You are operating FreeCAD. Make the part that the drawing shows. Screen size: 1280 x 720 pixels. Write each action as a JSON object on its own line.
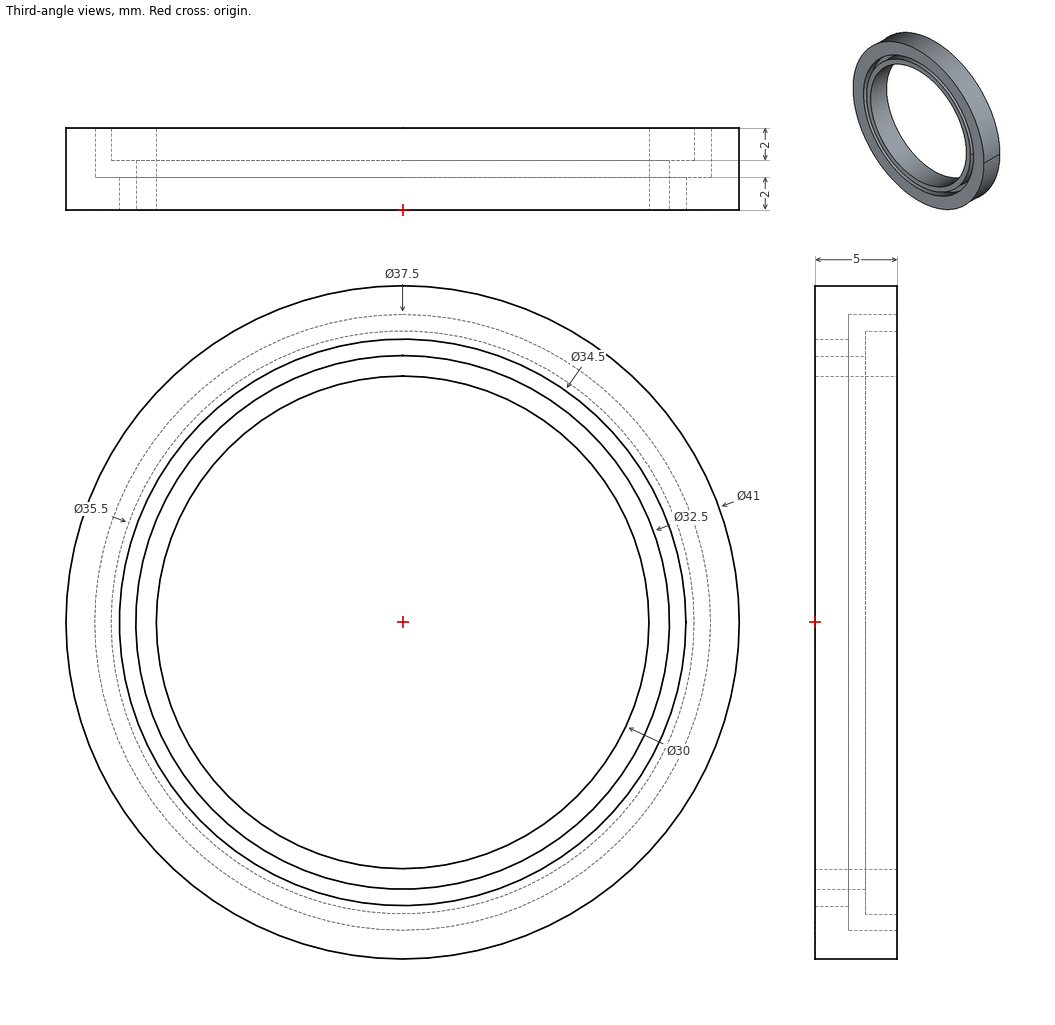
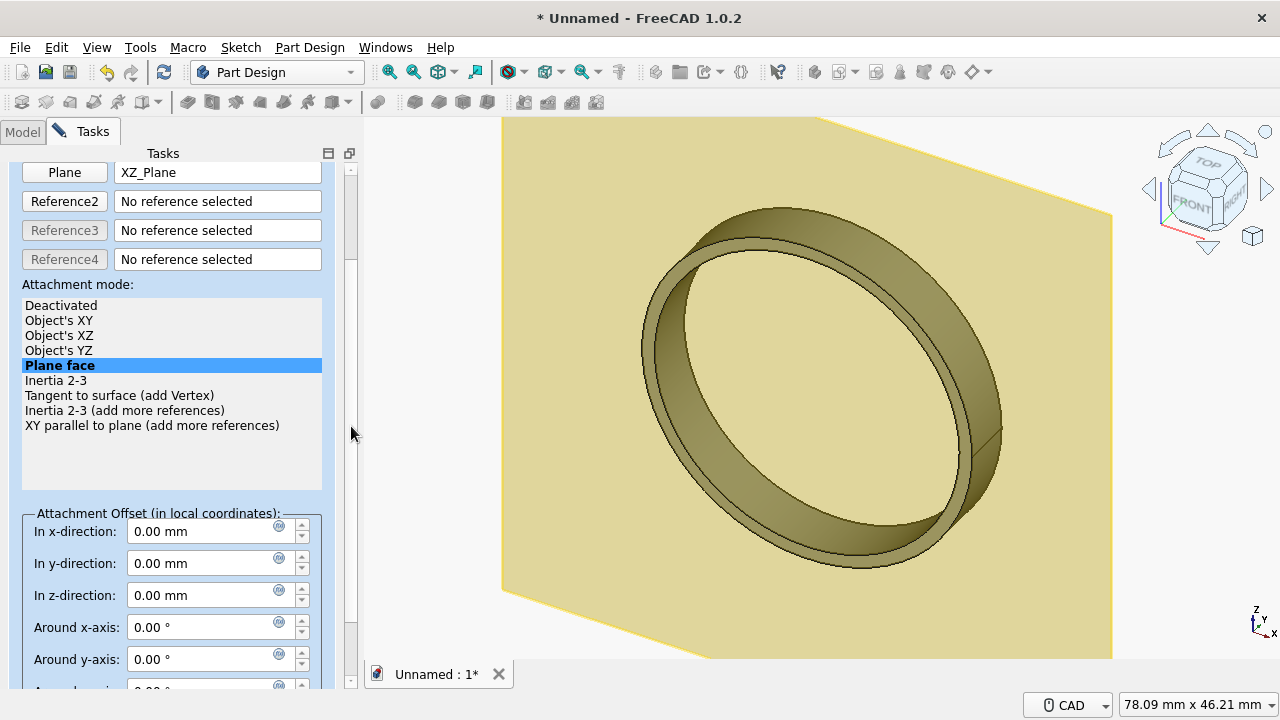
{"action": "triple_click", "coordinate": [210, 595]}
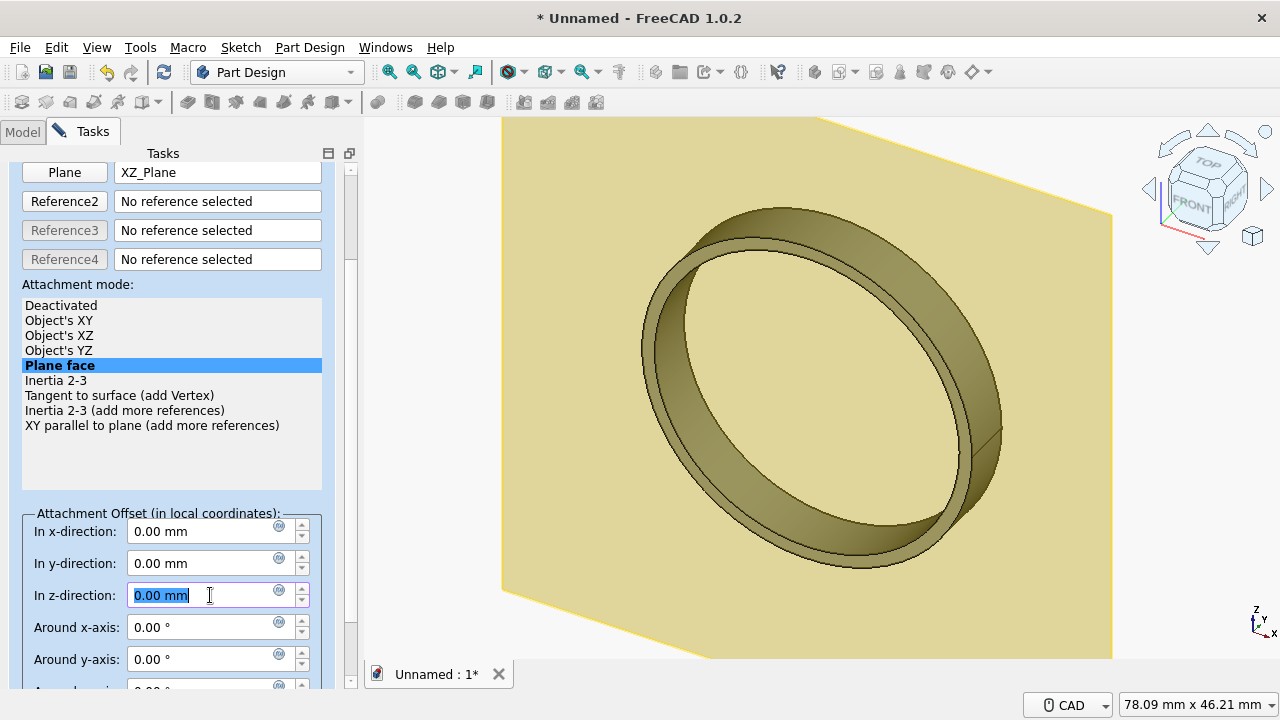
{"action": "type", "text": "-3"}
{"action": "key", "text": "Tab"}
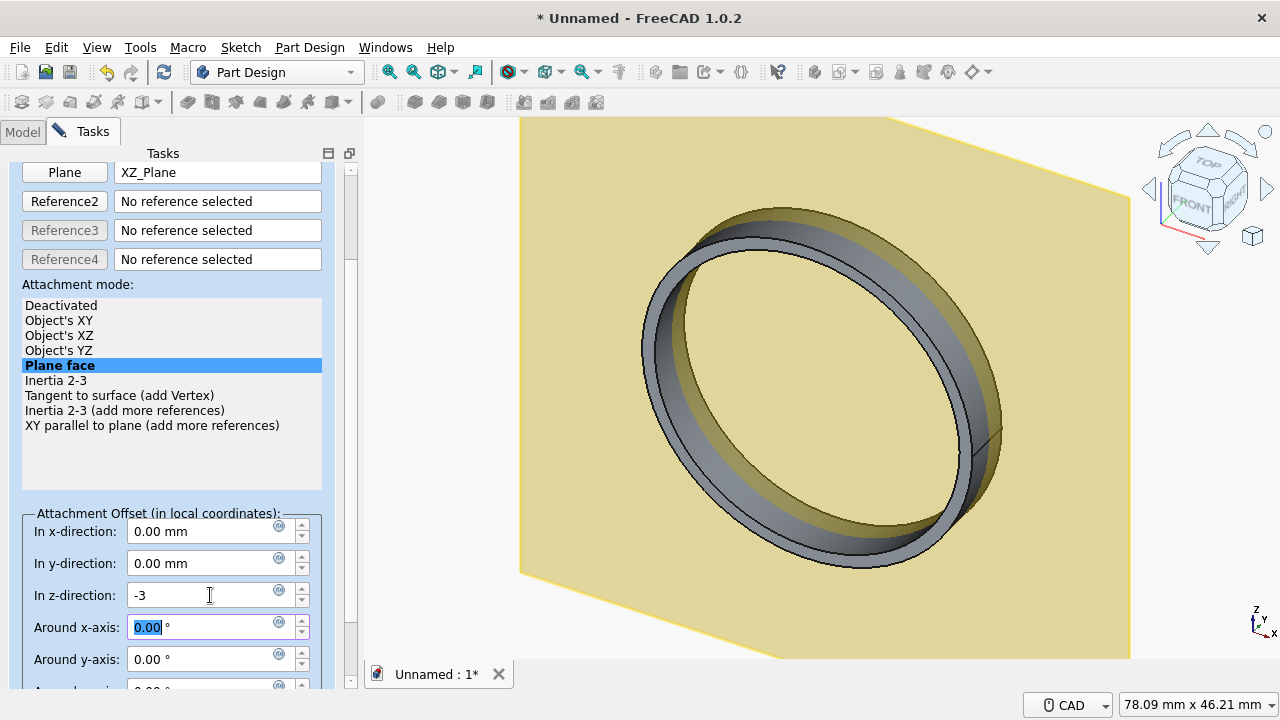
{"action": "scroll", "coordinate": [351, 426], "scroll_direction": "up", "scroll_amount": 3}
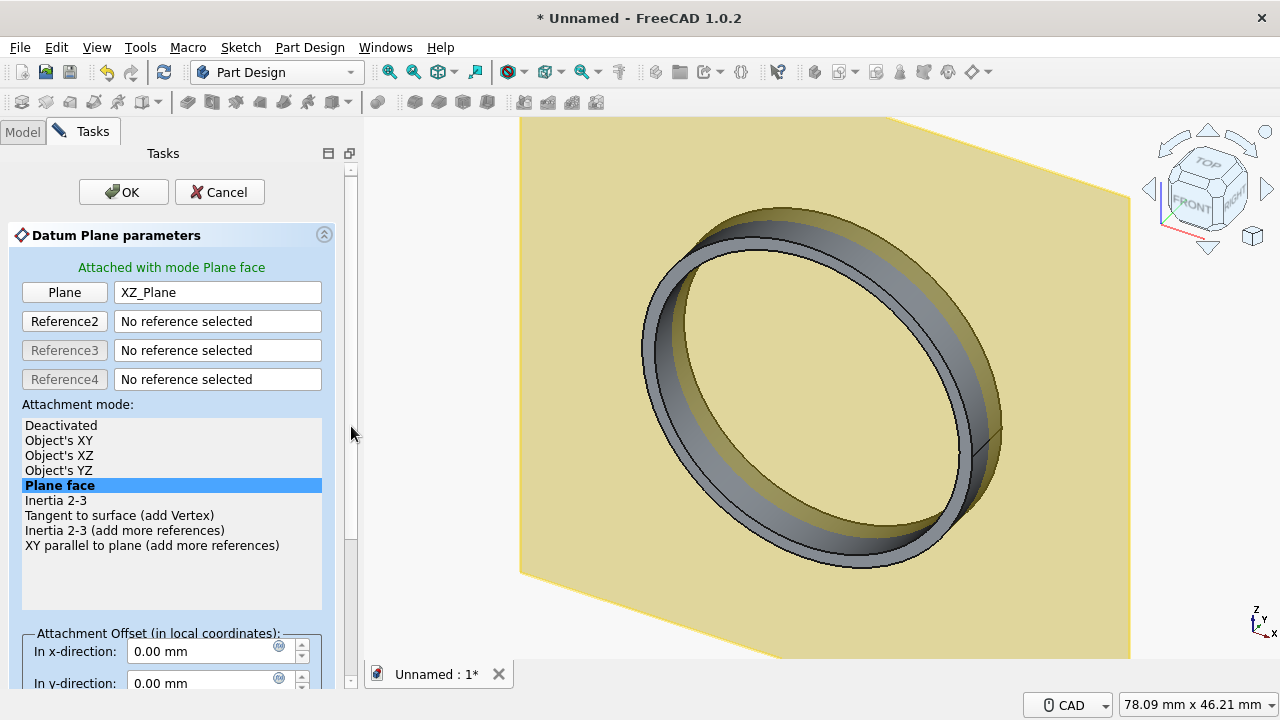
{"action": "left_click", "coordinate": [124, 192]}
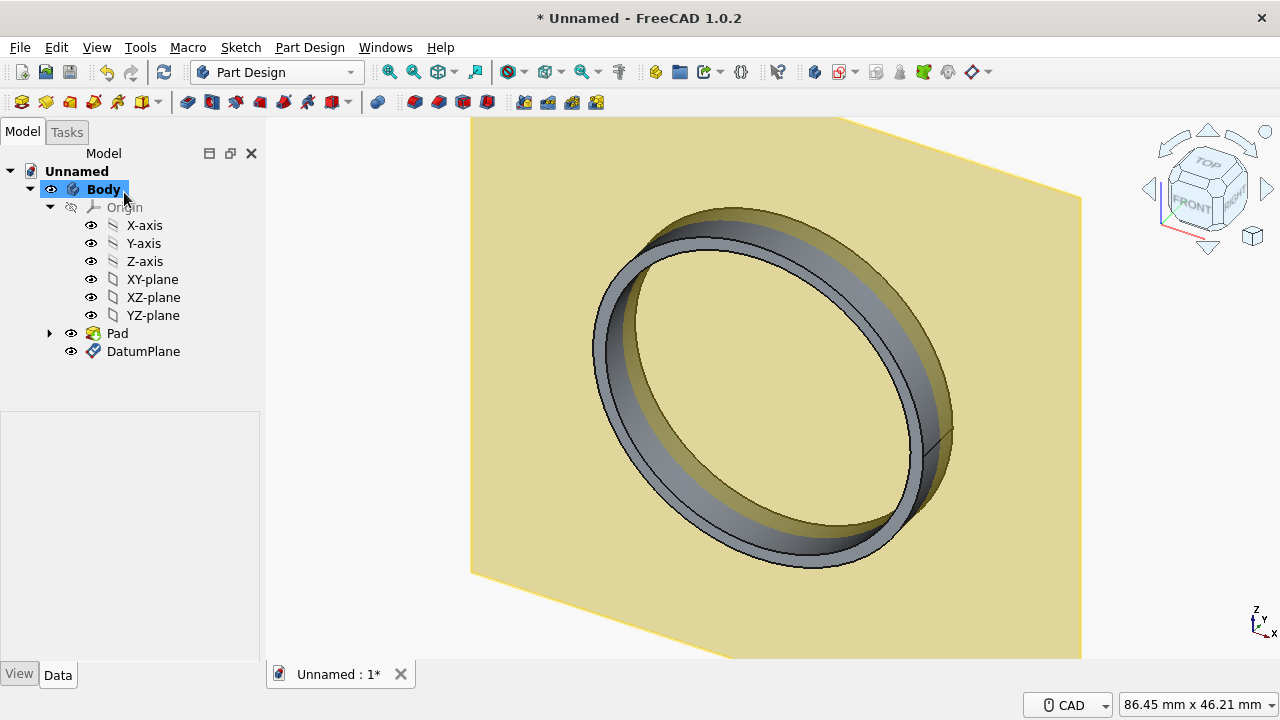
{"action": "left_click", "coordinate": [116, 351]}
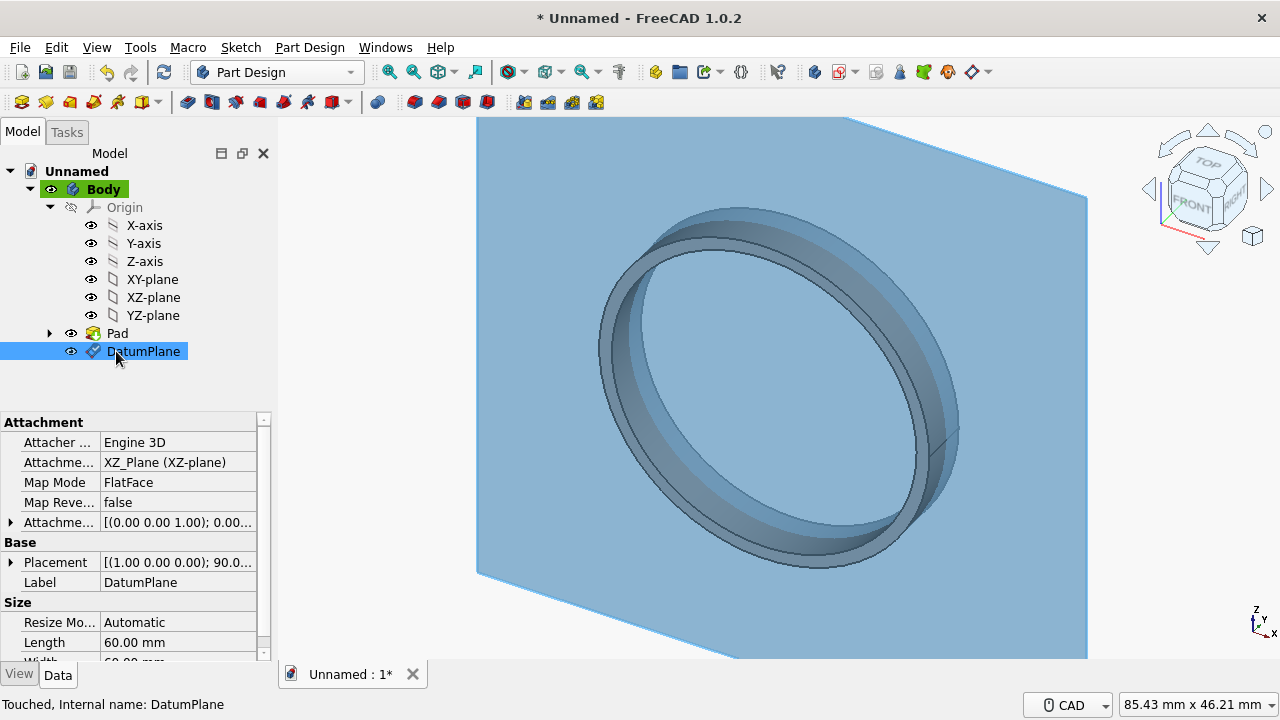
{"action": "left_click", "coordinate": [840, 72]}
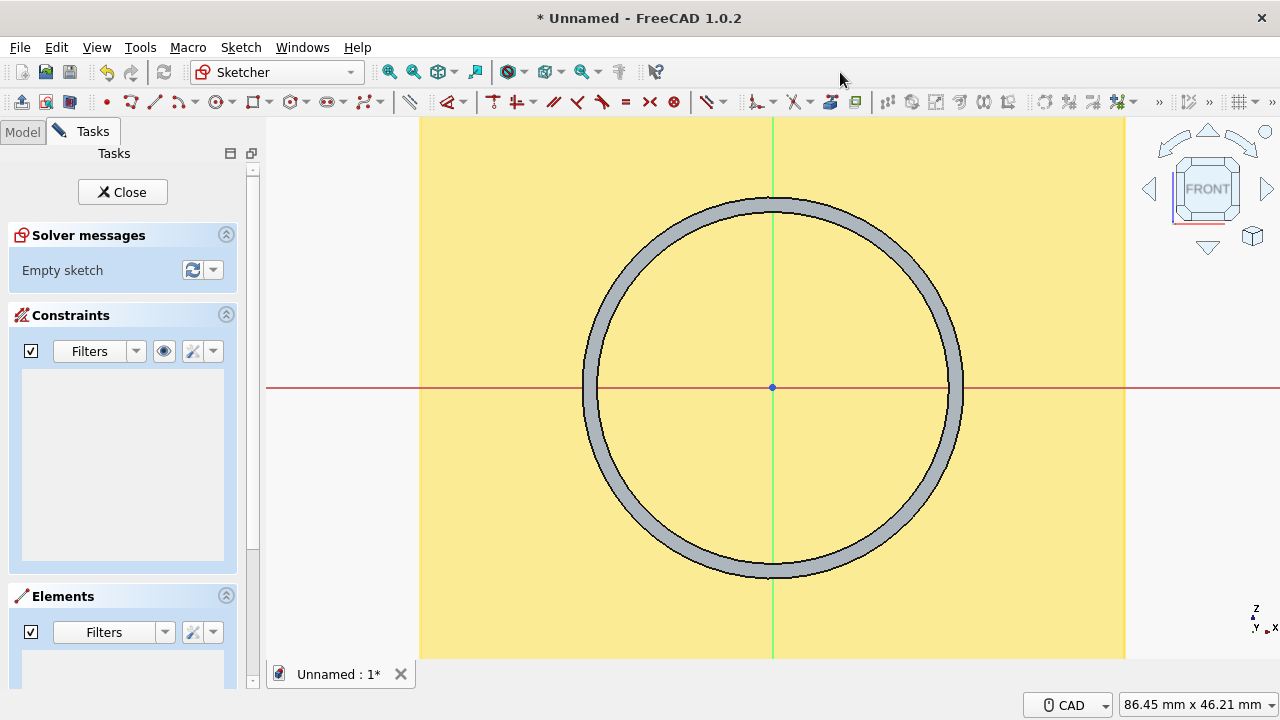
{"action": "key", "text": "q s"}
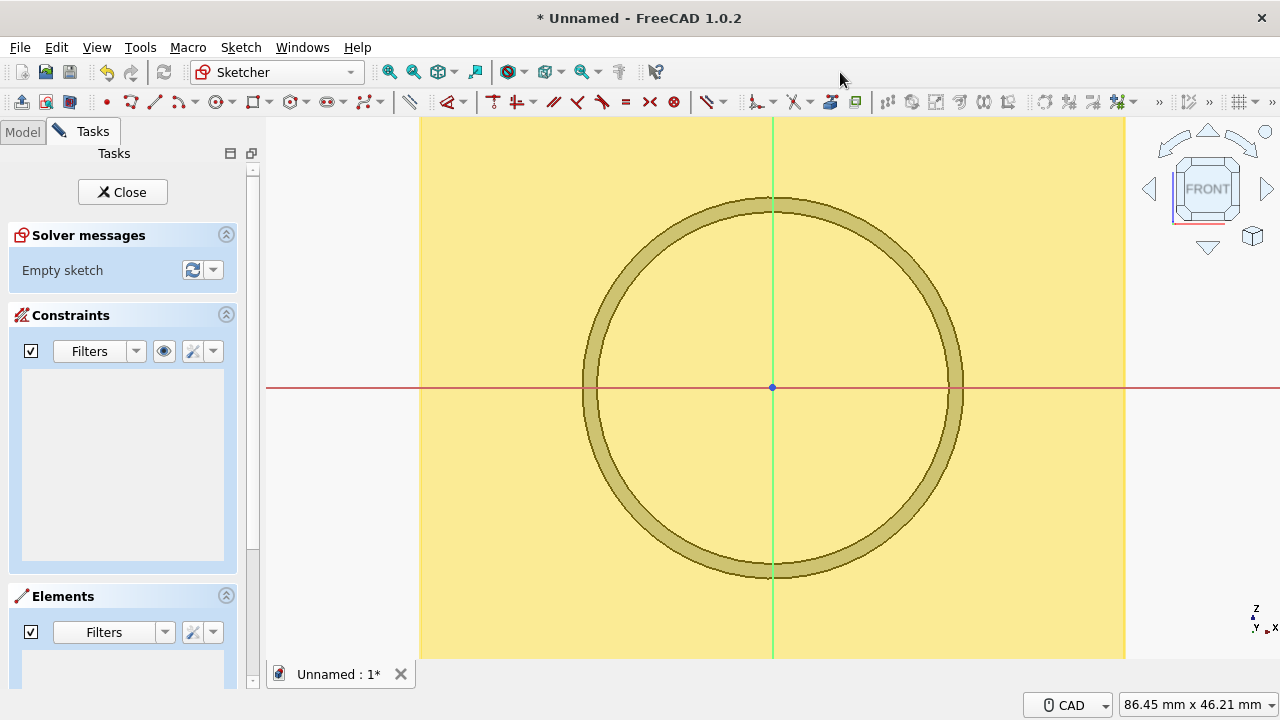
{"action": "key", "text": "g c"}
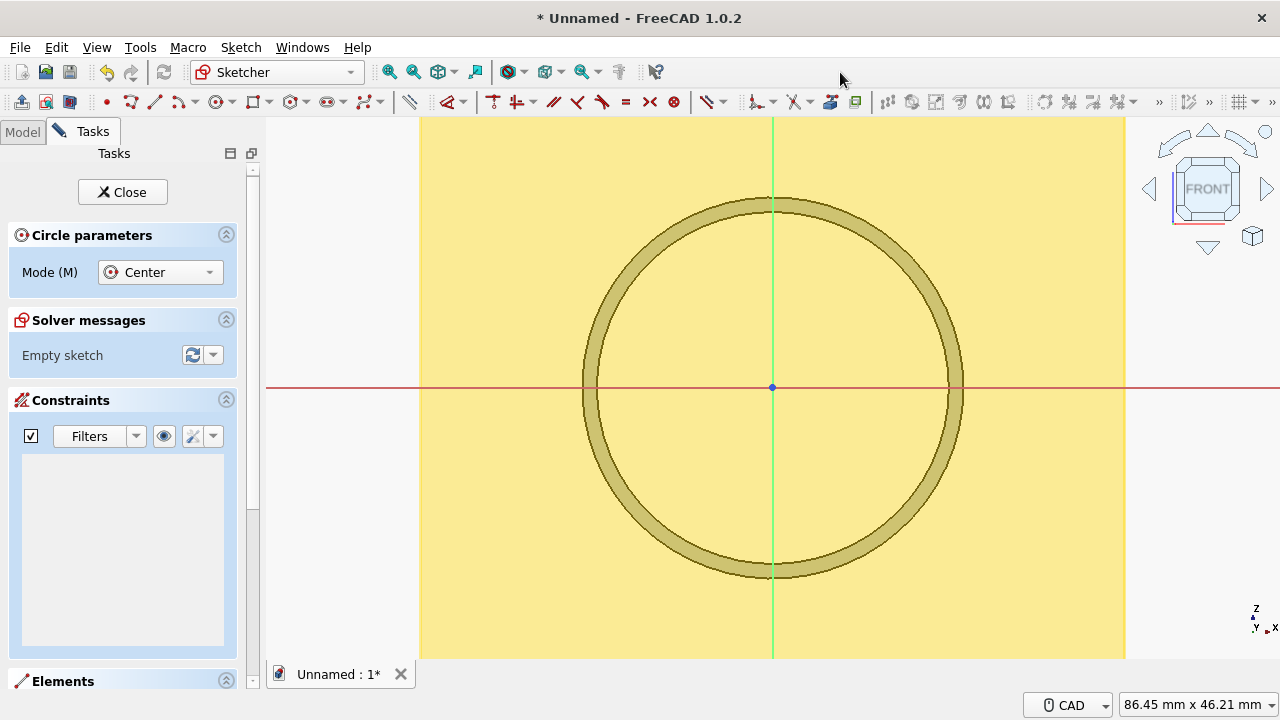
{"action": "left_click", "coordinate": [773, 388]}
{"action": "mouse_move", "coordinate": [920, 241]}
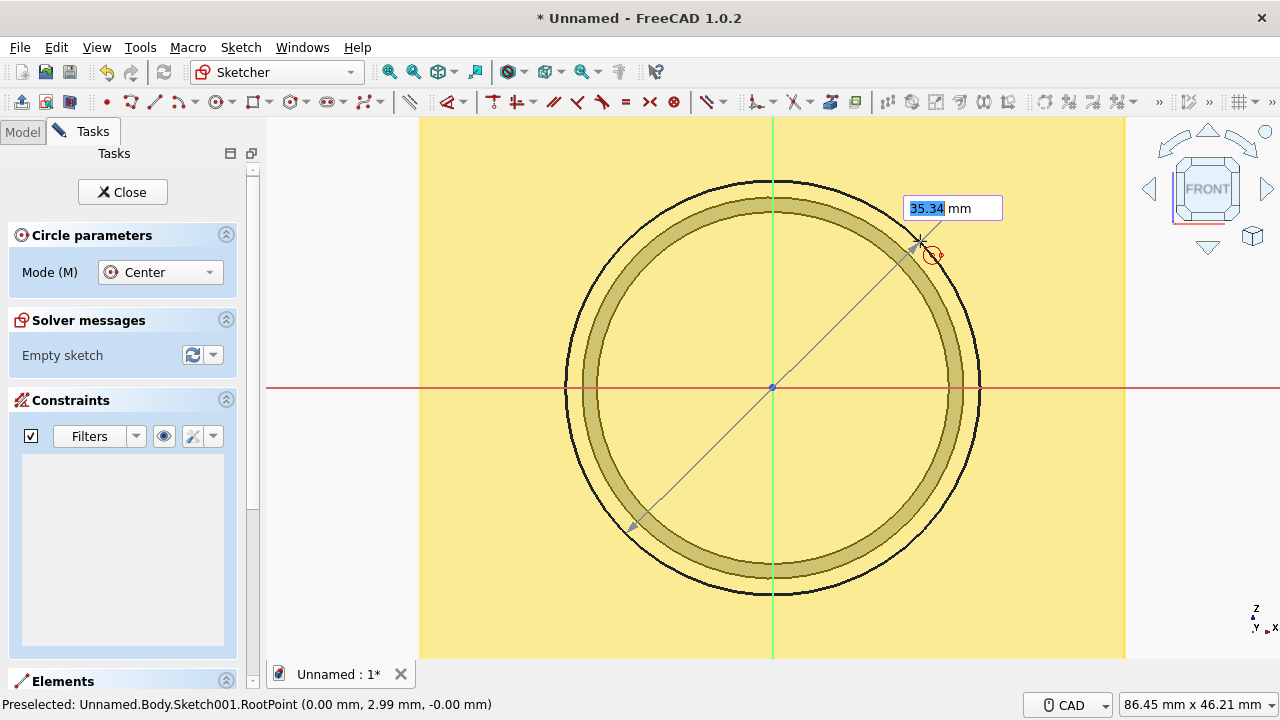
{"action": "type", "text": "35.5"}
{"action": "key", "text": "Return"}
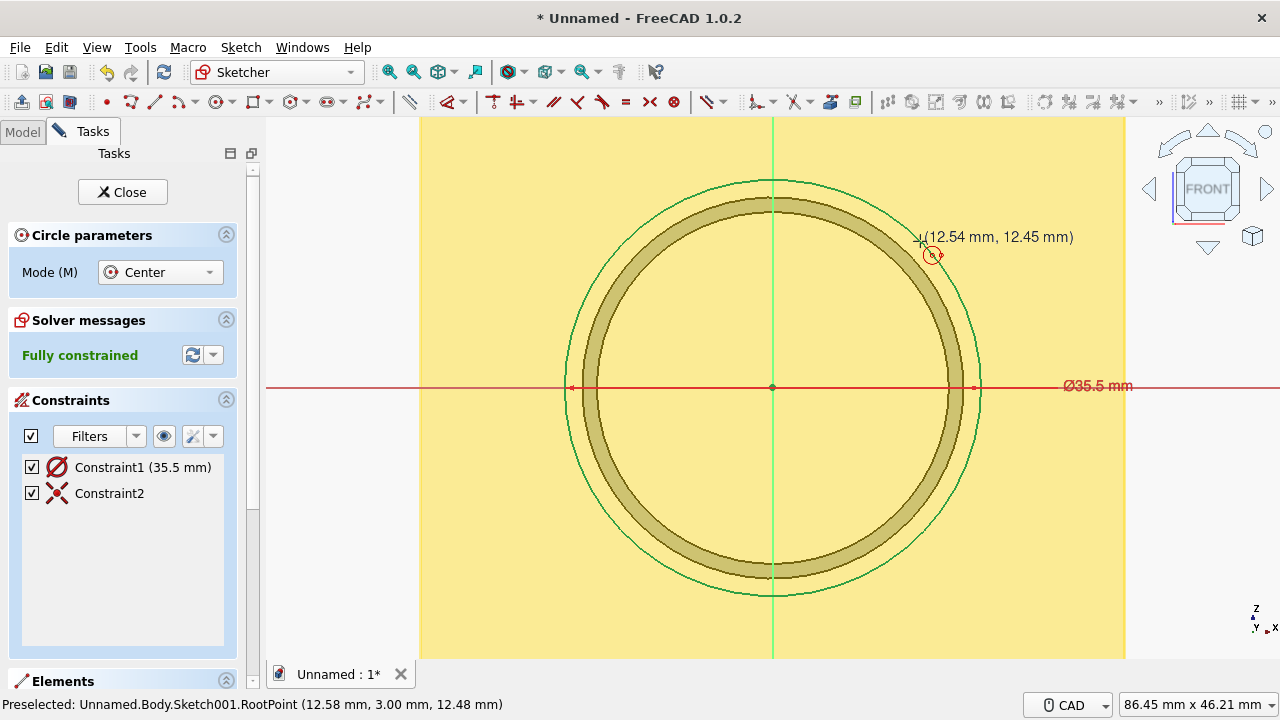
{"action": "left_click", "coordinate": [773, 388]}
{"action": "mouse_move", "coordinate": [908, 253]}